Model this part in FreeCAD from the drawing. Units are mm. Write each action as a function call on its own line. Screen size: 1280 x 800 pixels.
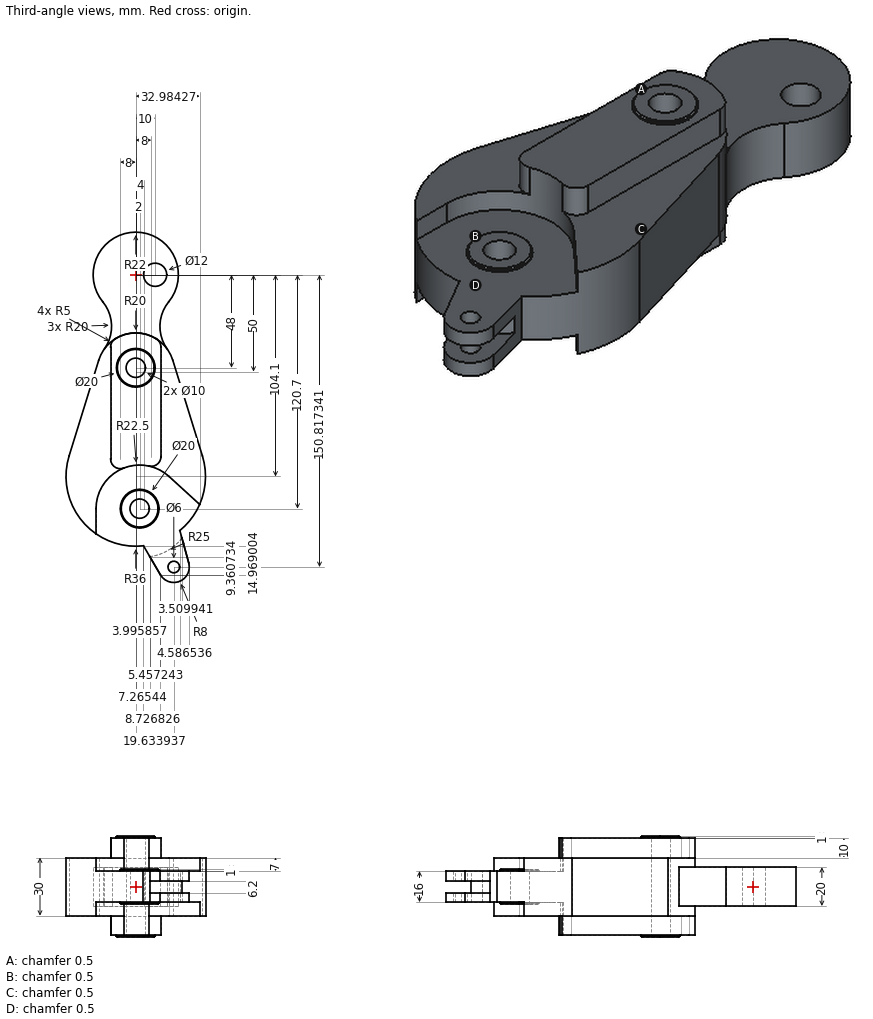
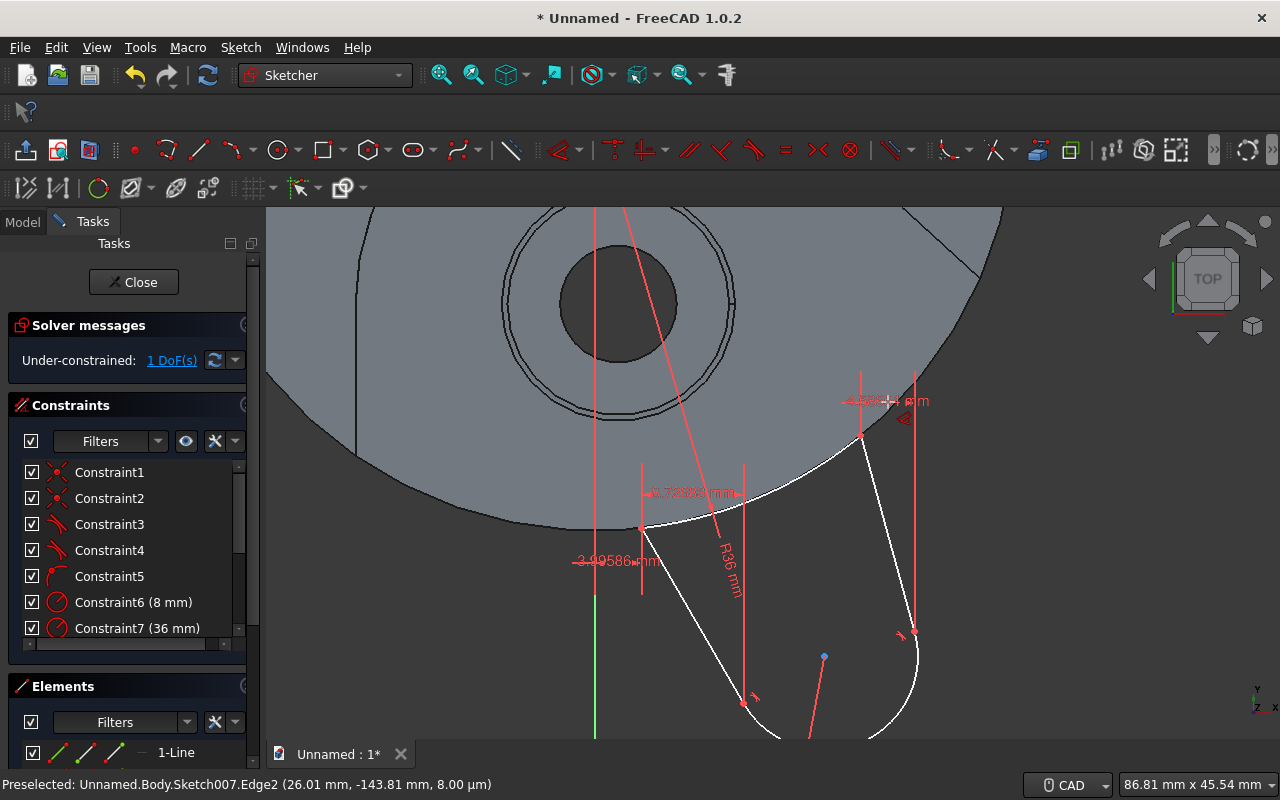
click(672, 581)
click(778, 616)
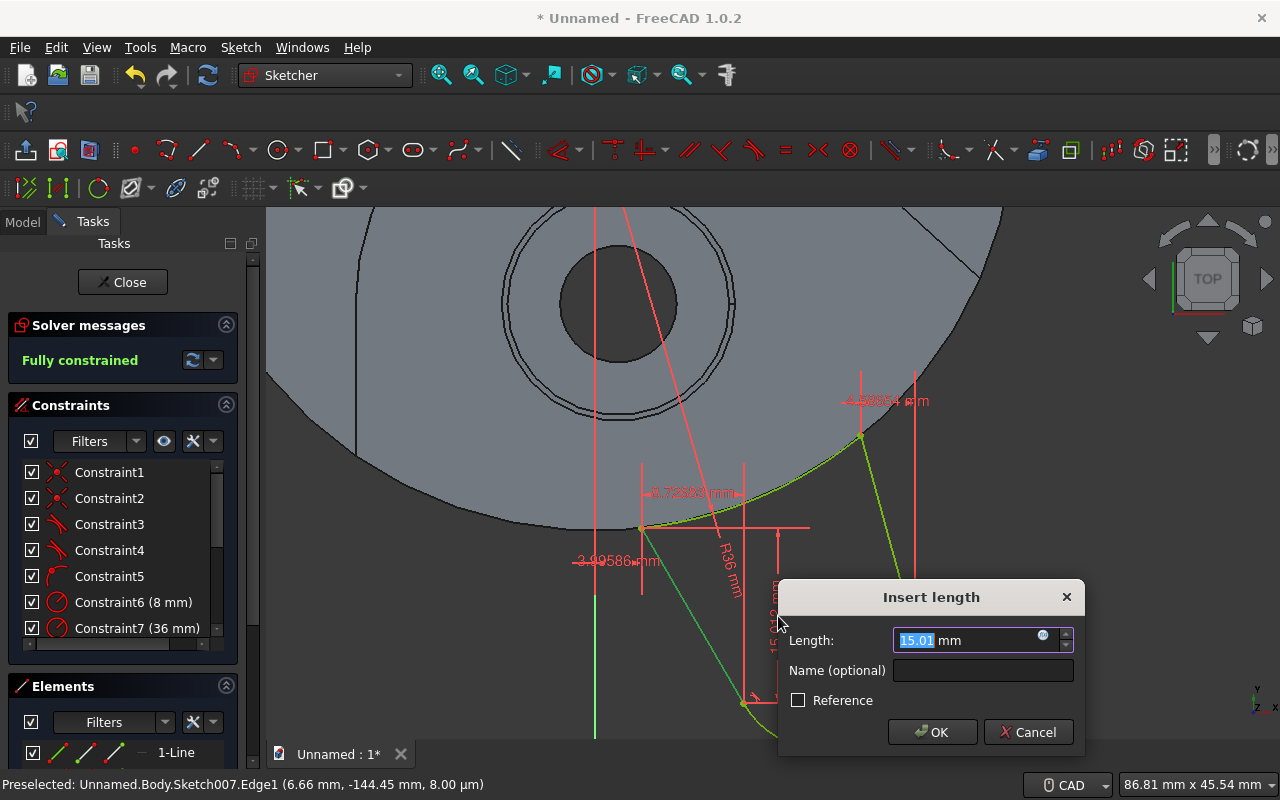
text(14.969004)
key(Return)
key(Escape)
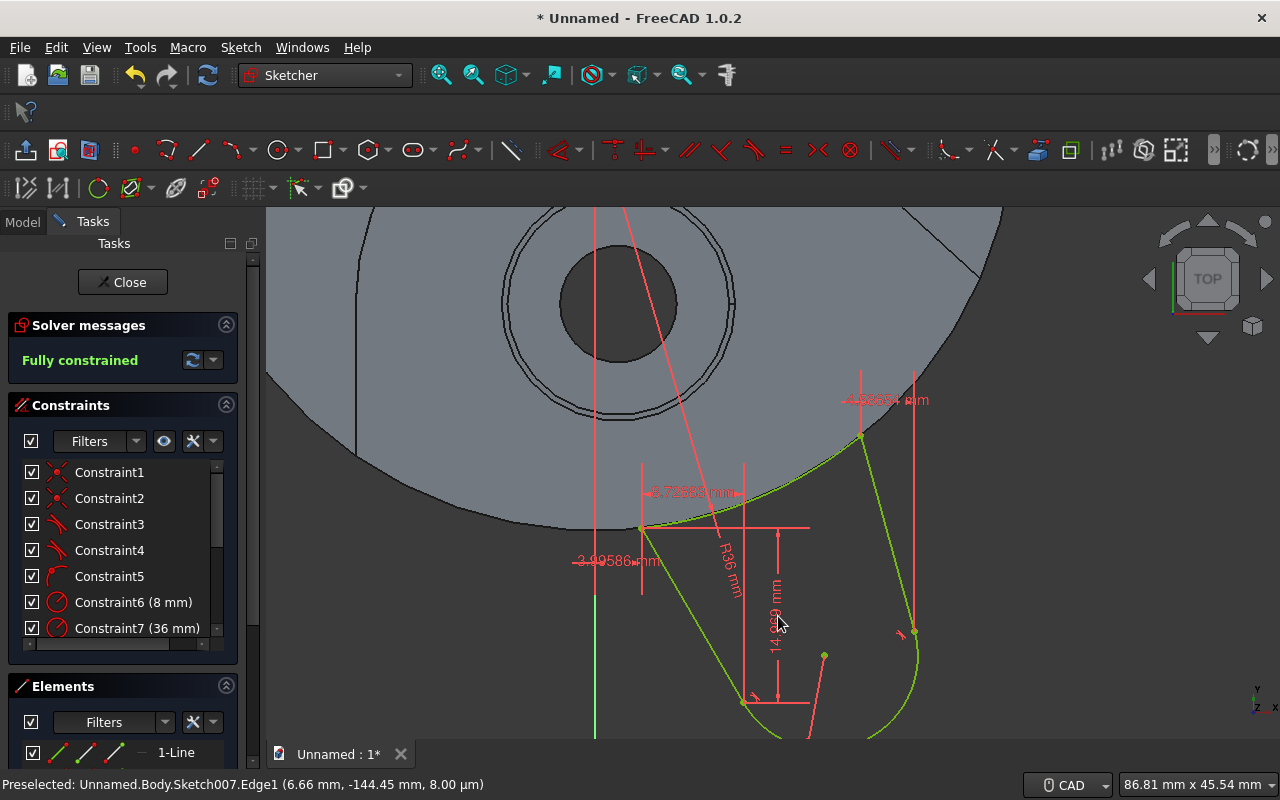
click(123, 282)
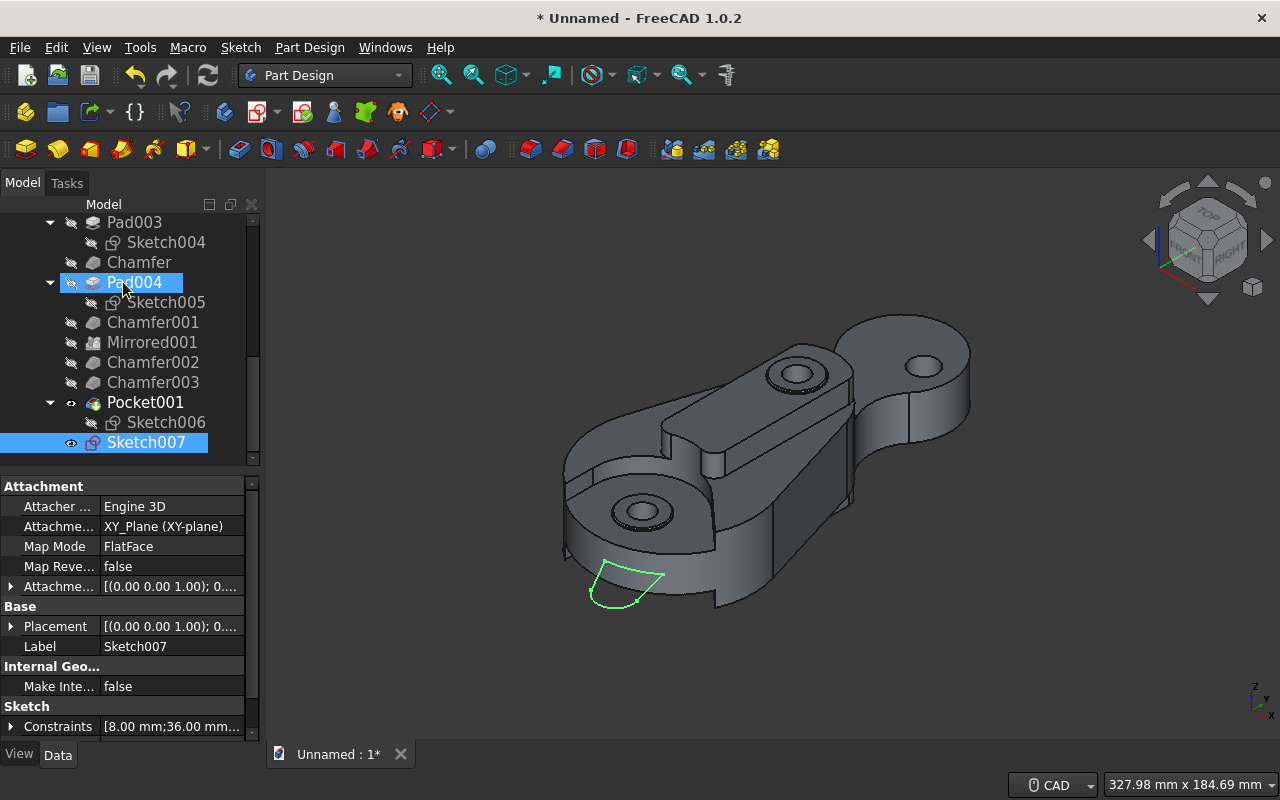
click(26, 150)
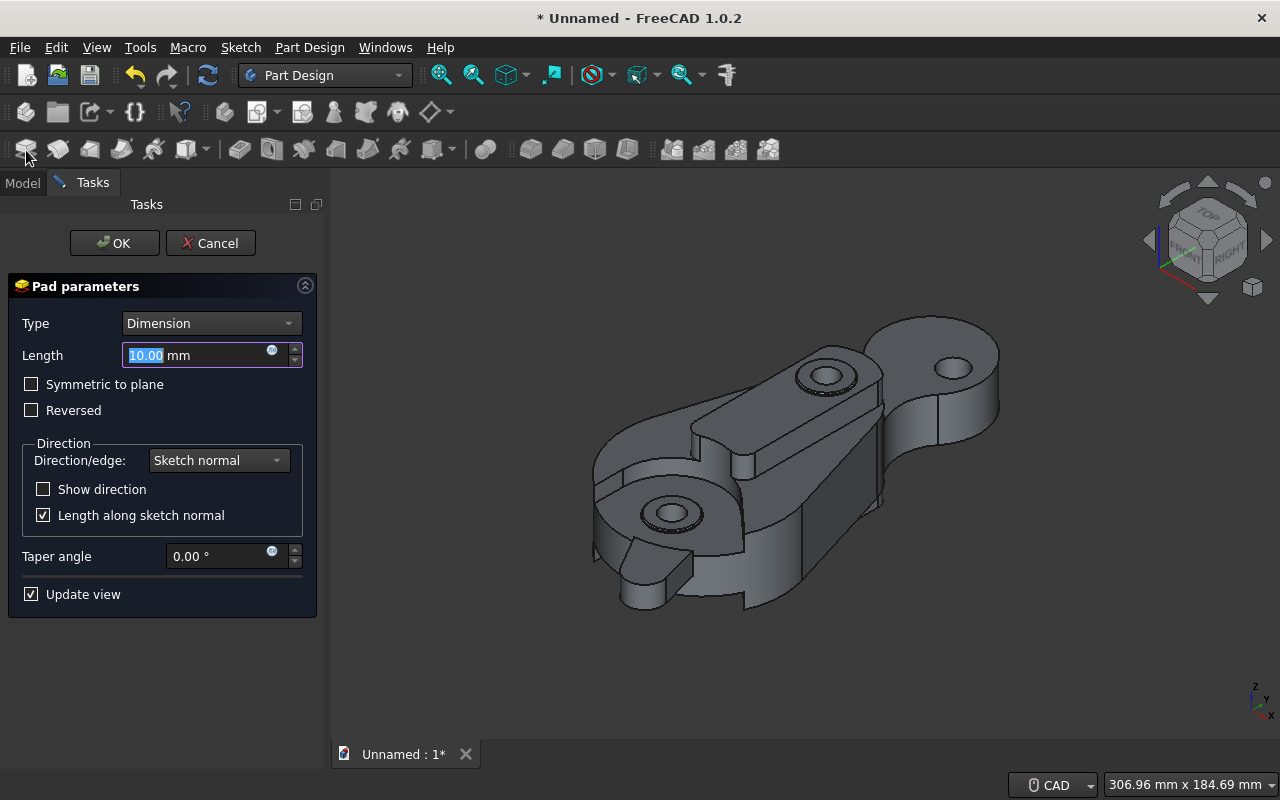
text(16)
key(Tab)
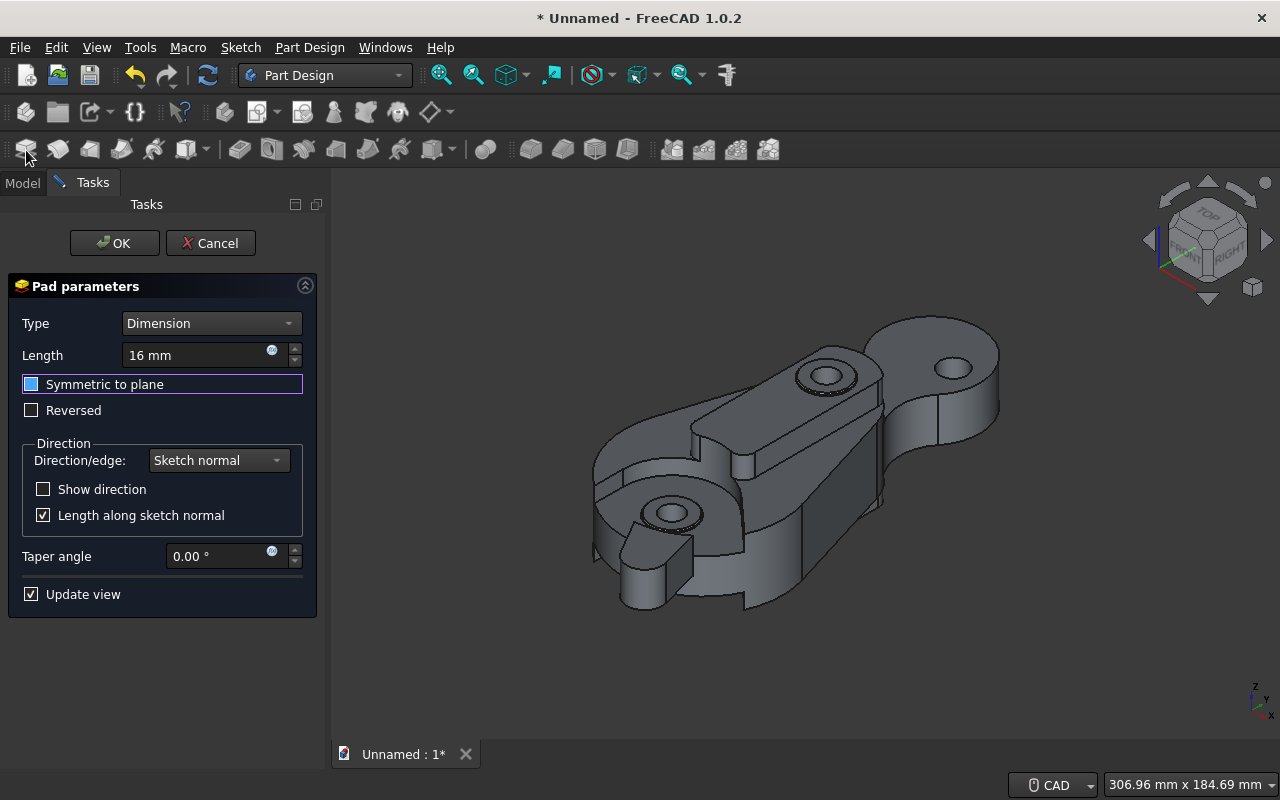
click(30, 384)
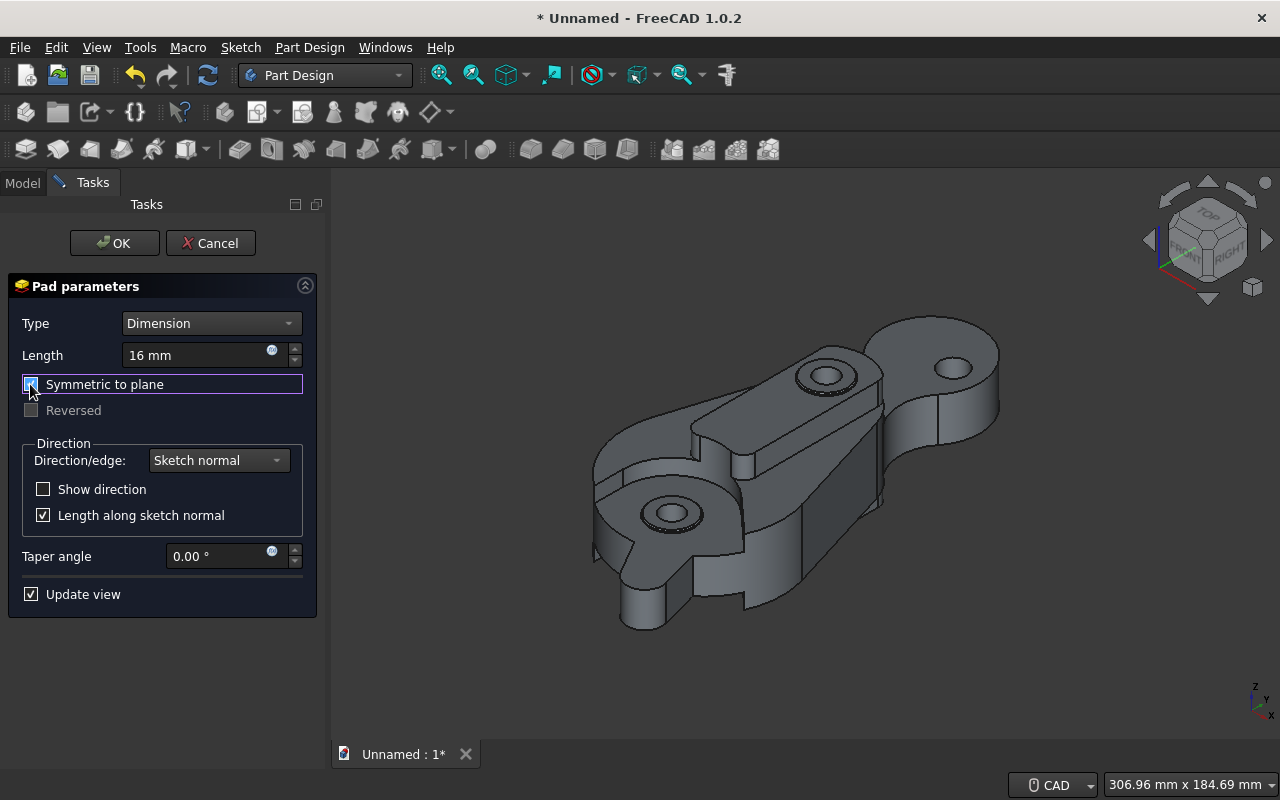
click(115, 243)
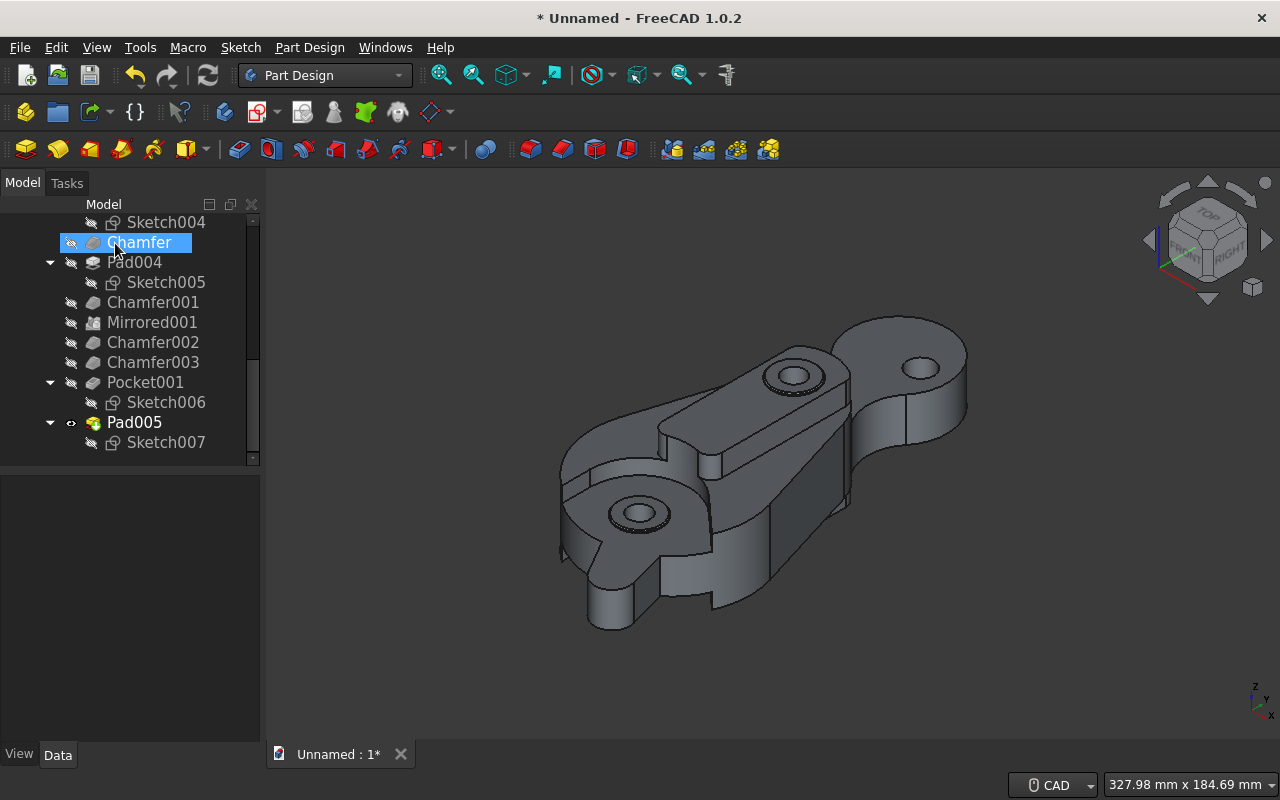
click(258, 112)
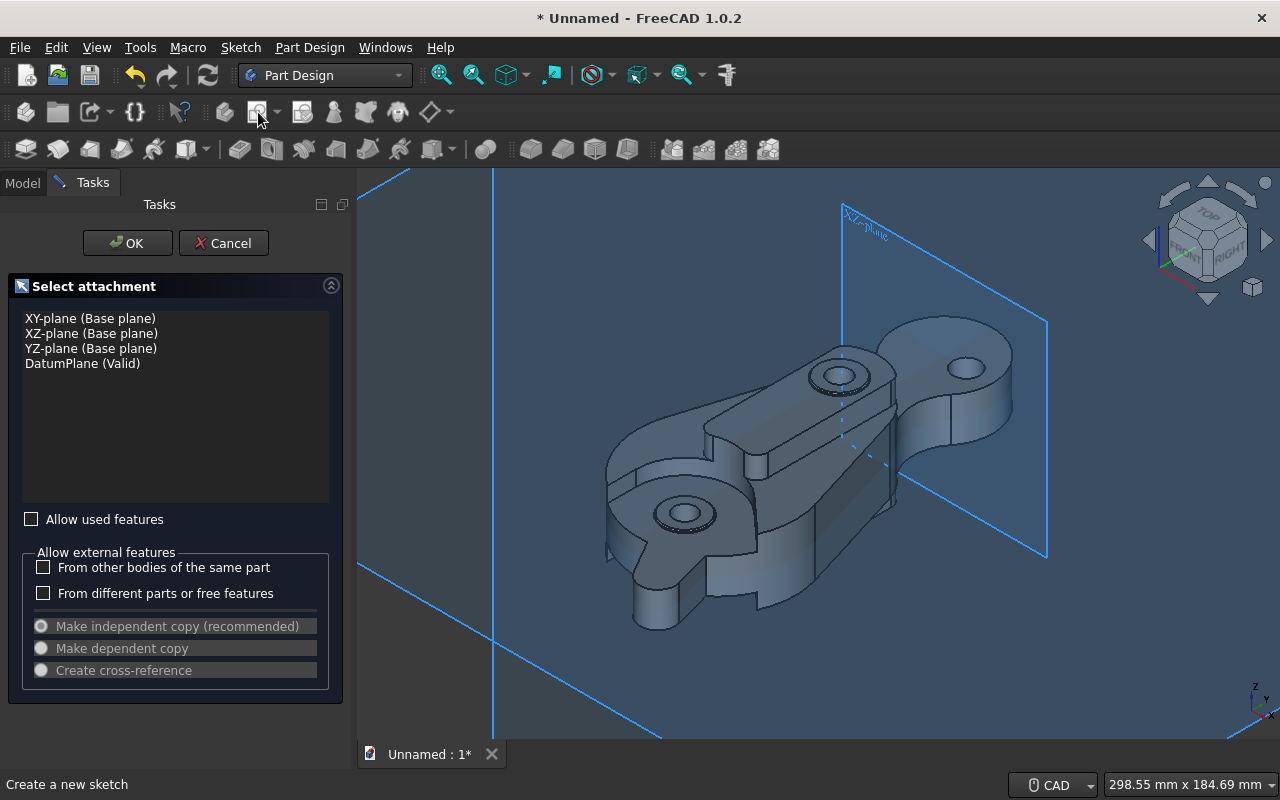
click(82, 318)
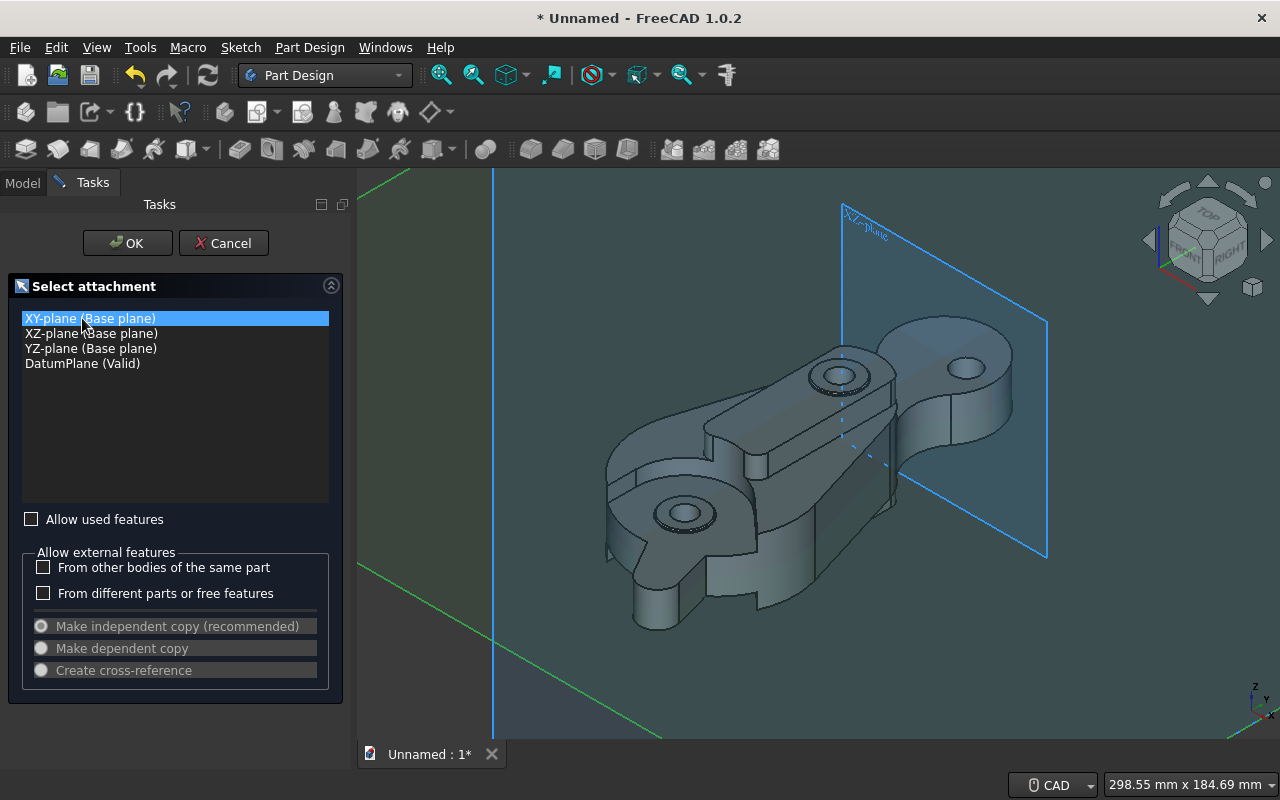
click(128, 243)